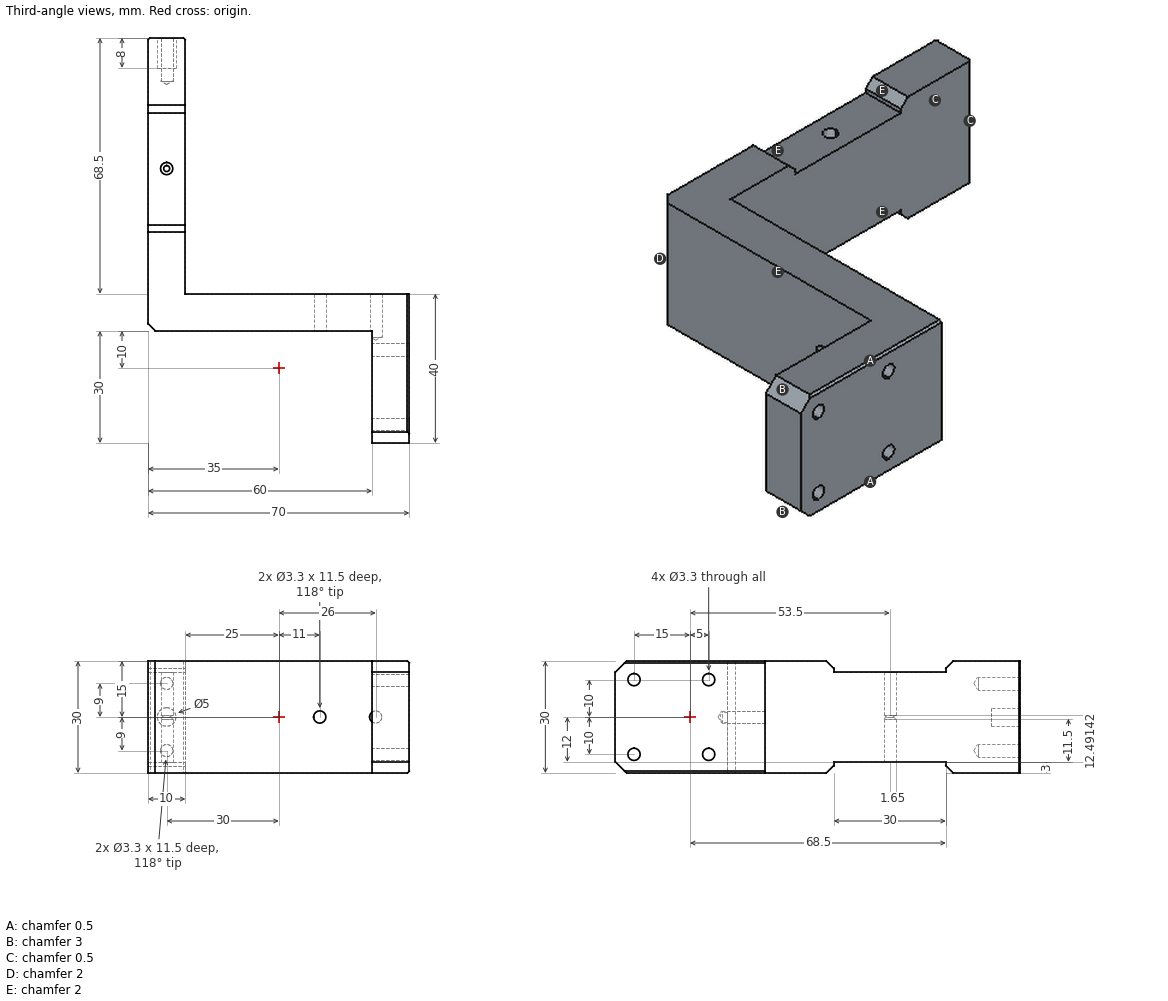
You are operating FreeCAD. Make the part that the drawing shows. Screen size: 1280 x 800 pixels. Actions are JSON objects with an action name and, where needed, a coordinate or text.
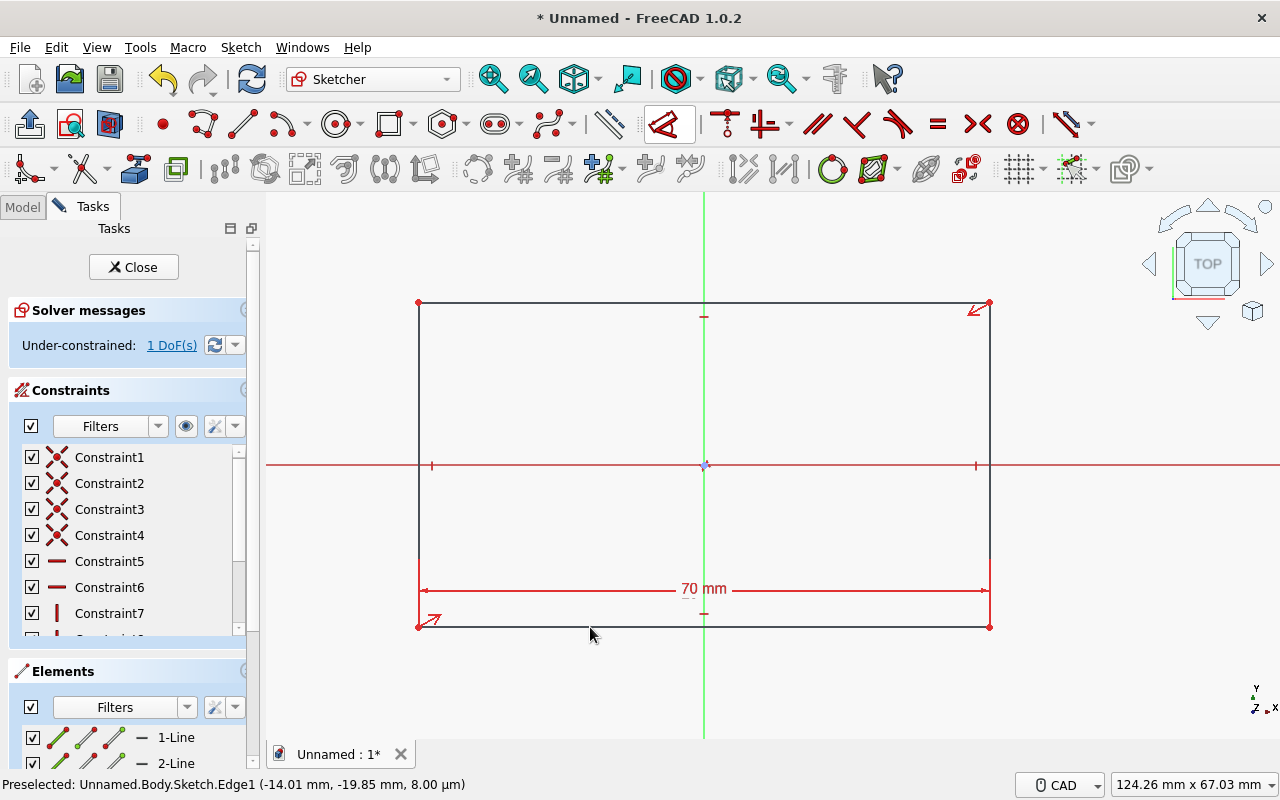
{"action": "left_click", "coordinate": [990, 530]}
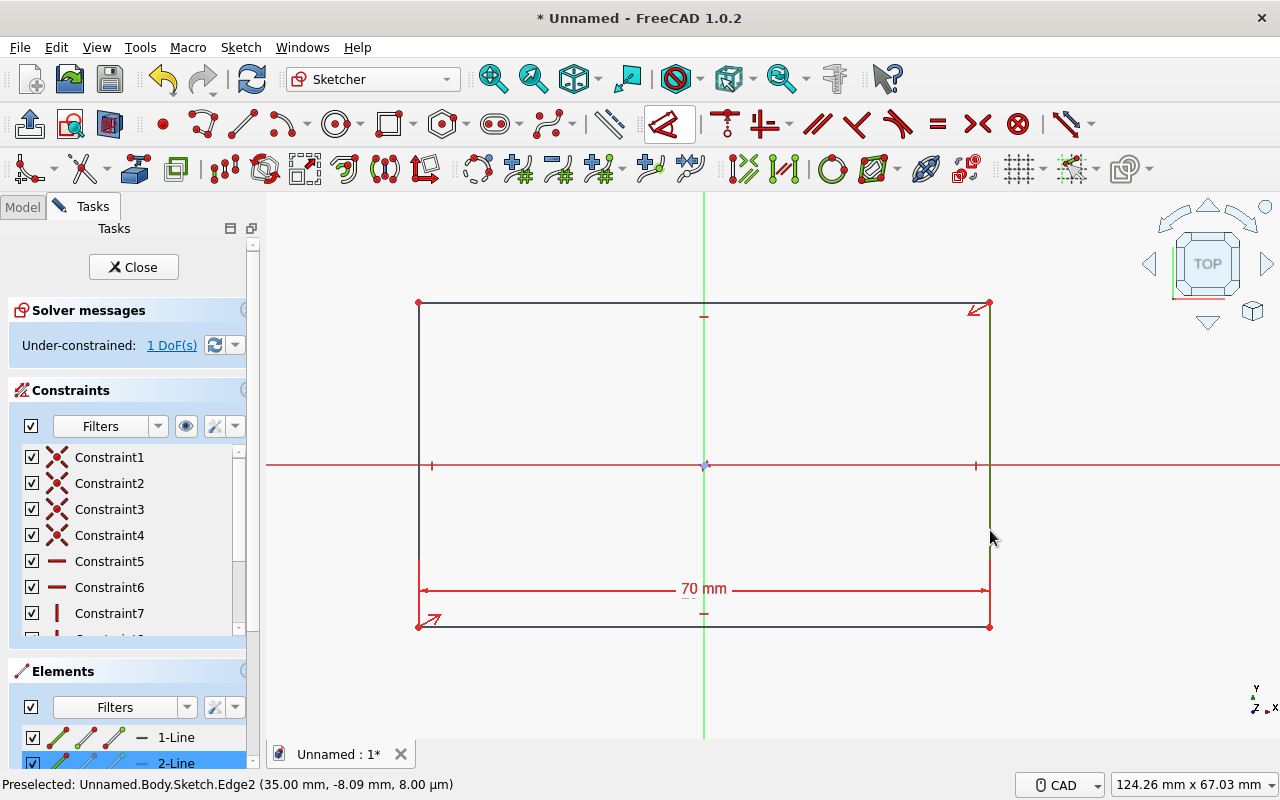
{"action": "key", "text": "i"}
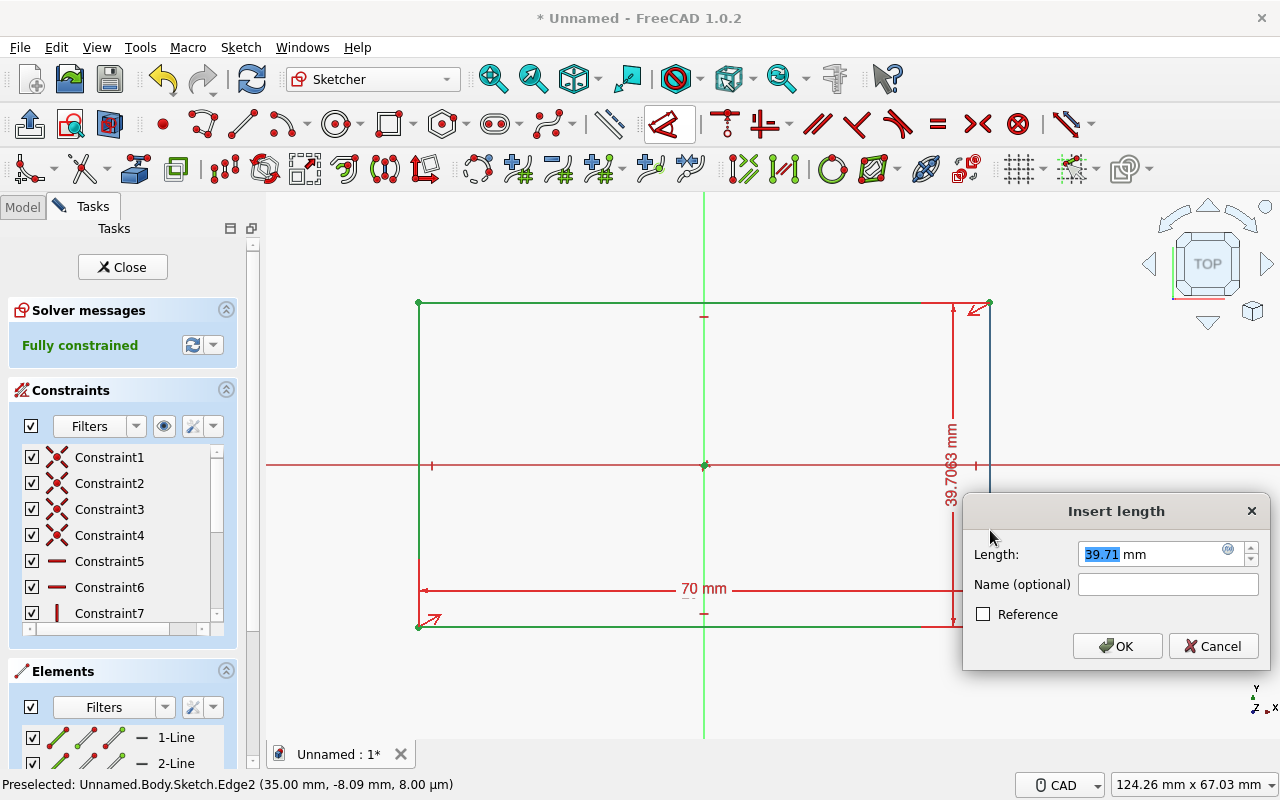
{"action": "type", "text": "40"}
{"action": "key", "text": "Return"}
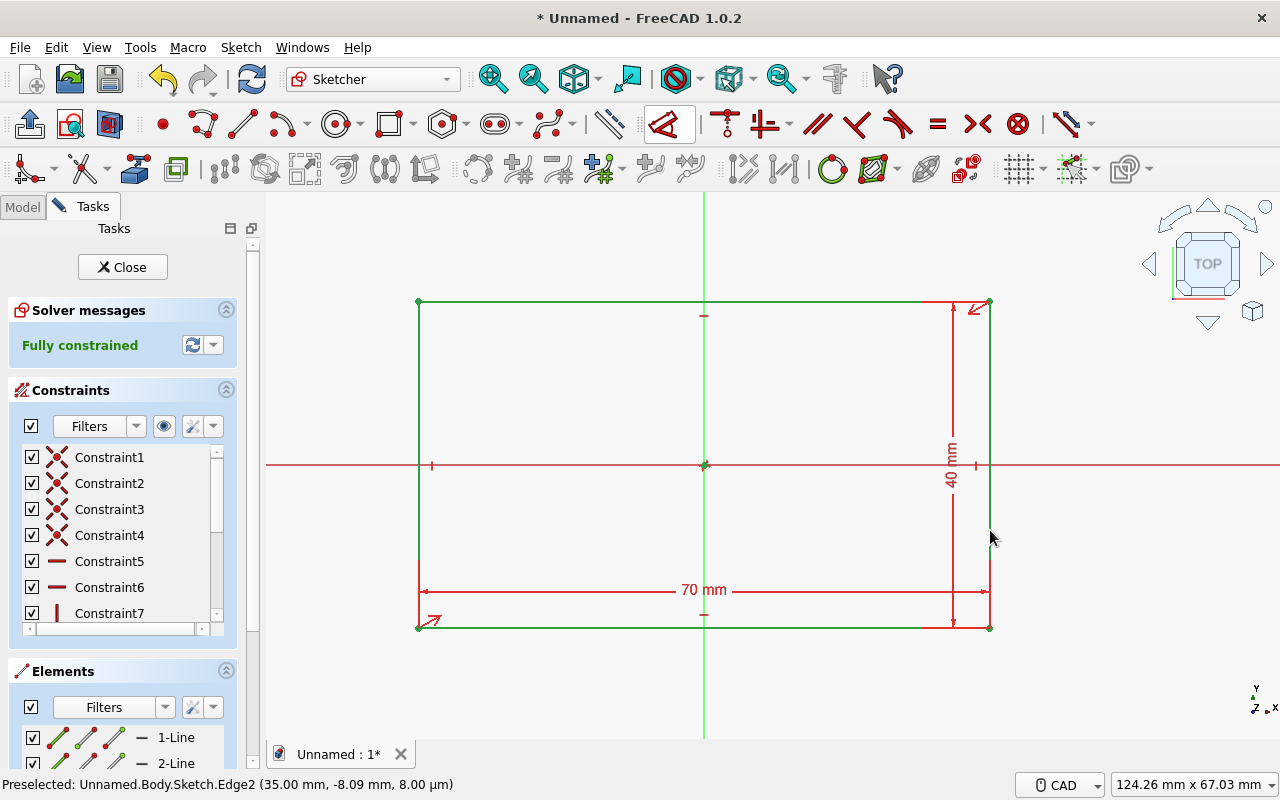
{"action": "left_click", "coordinate": [123, 267]}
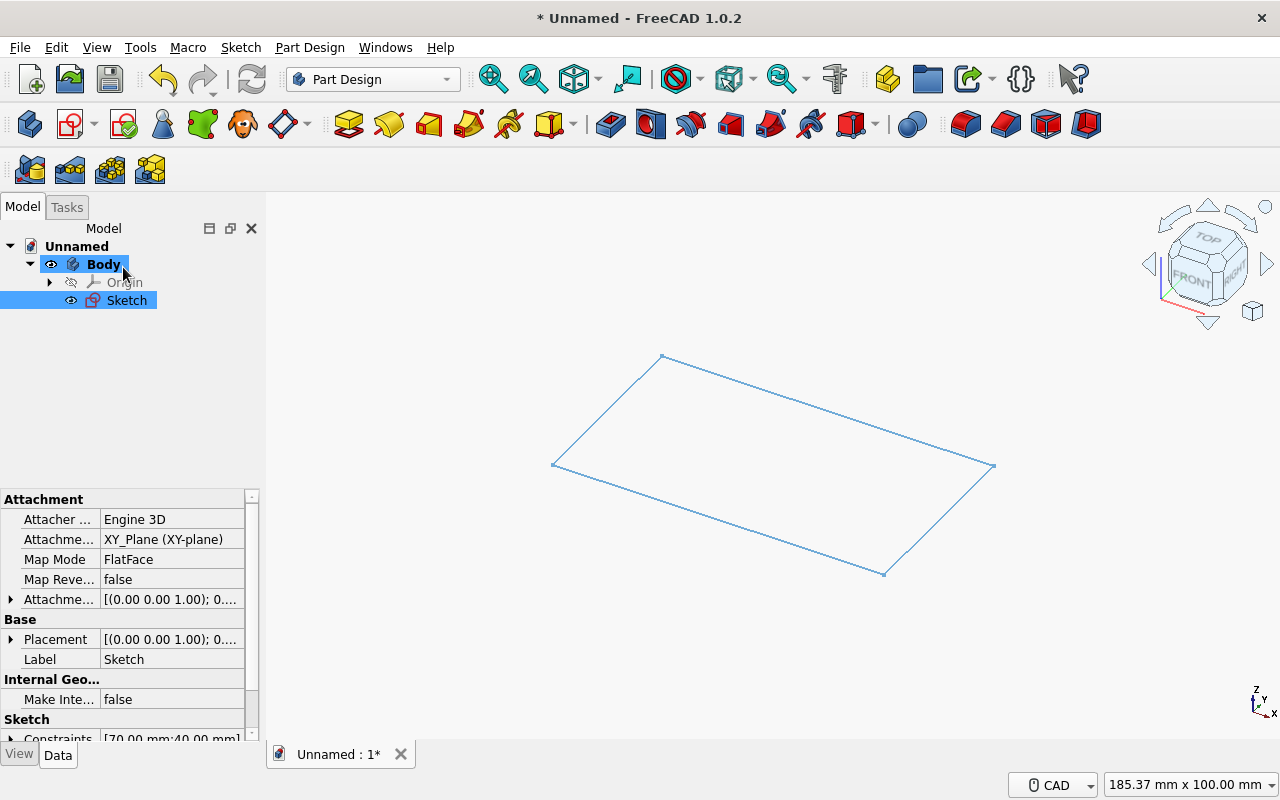
{"action": "left_click", "coordinate": [350, 124]}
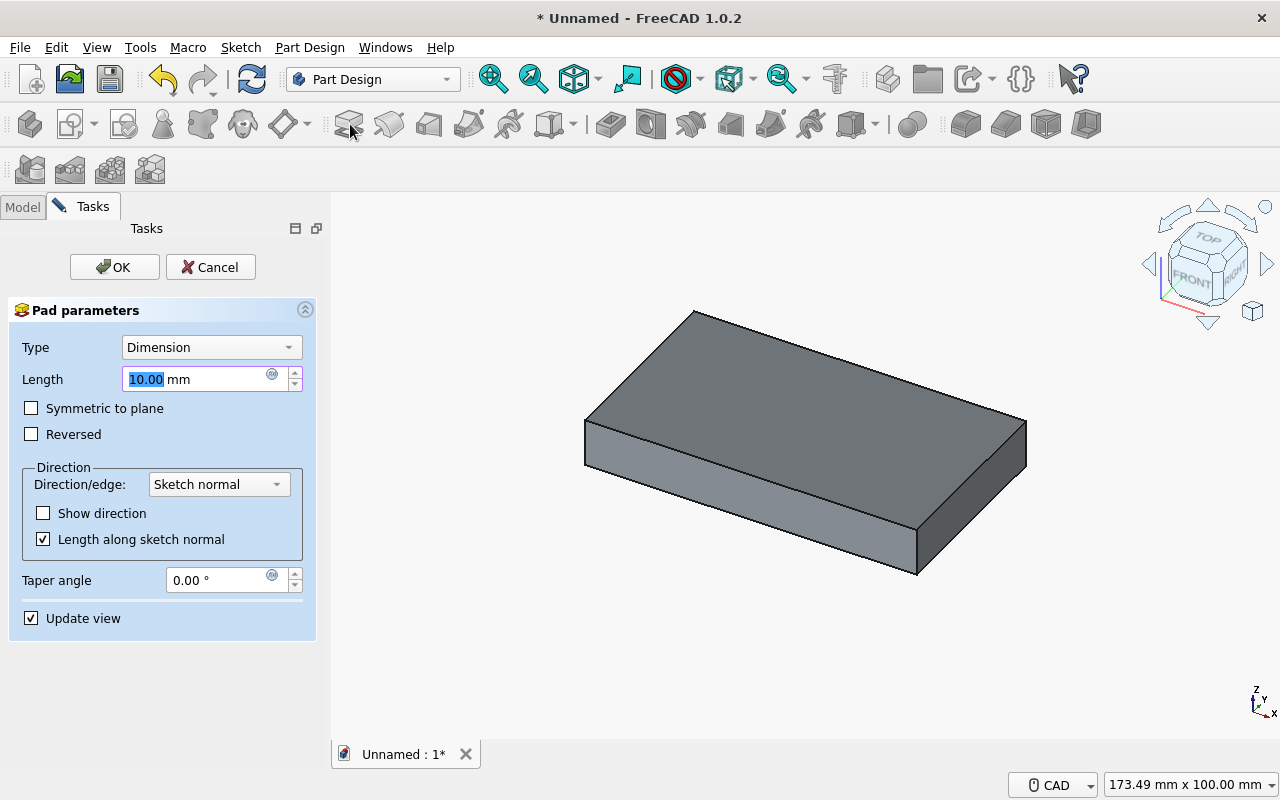
{"action": "type", "text": "30"}
{"action": "key", "text": "Tab"}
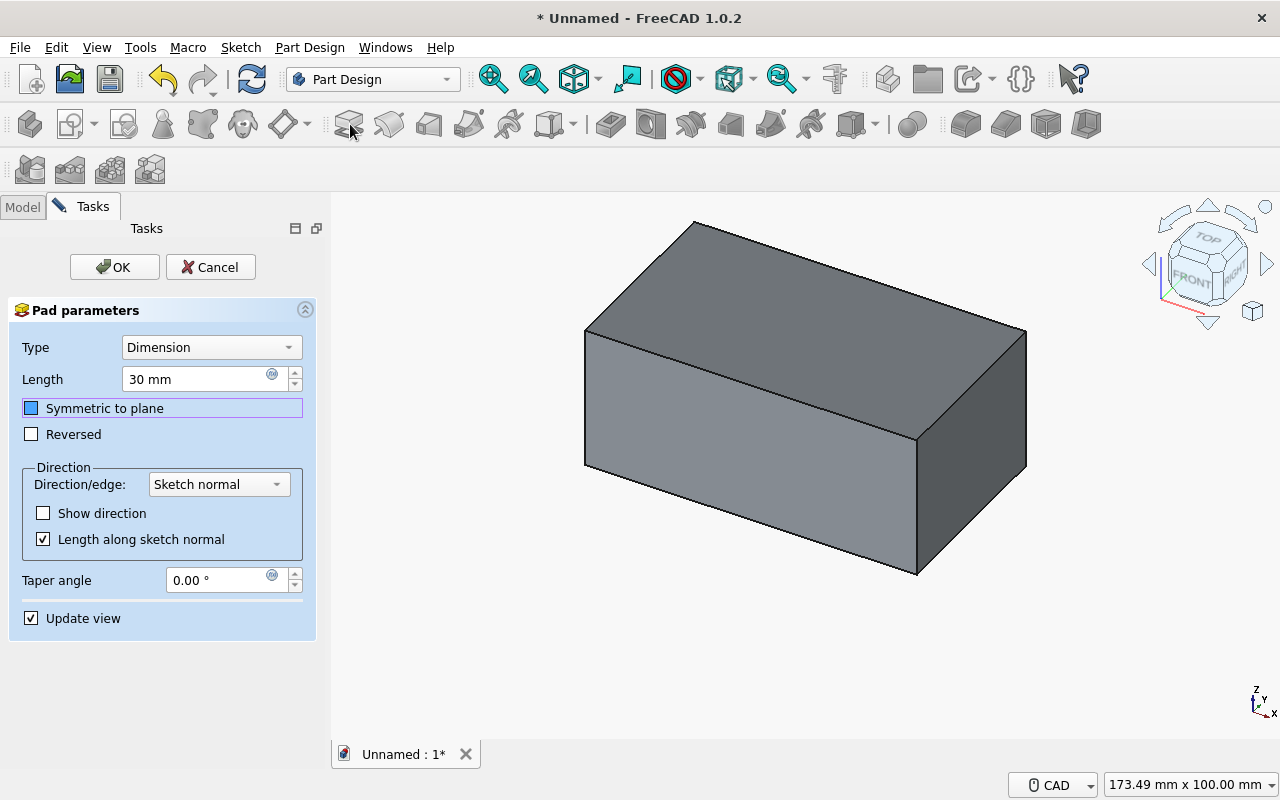
{"action": "left_click", "coordinate": [30, 408]}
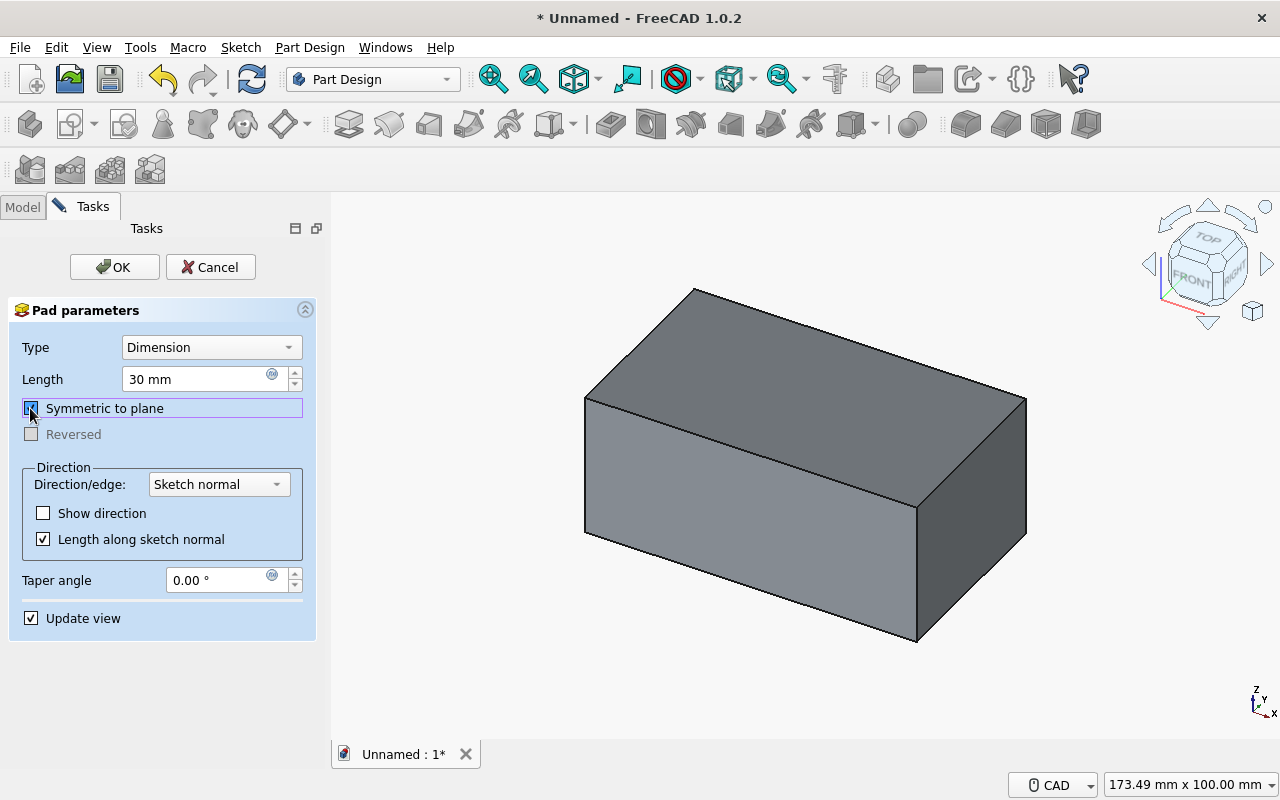
{"action": "left_click", "coordinate": [115, 267]}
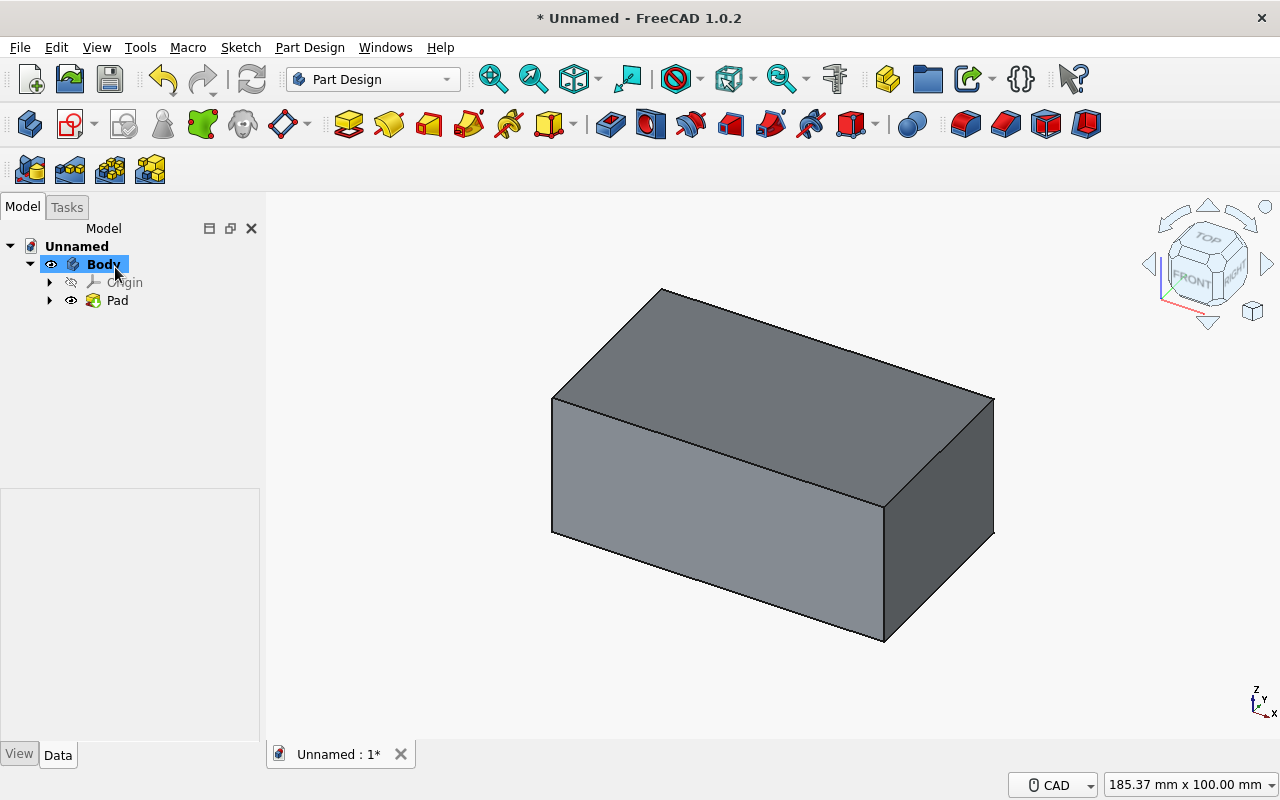
{"action": "left_click", "coordinate": [820, 413]}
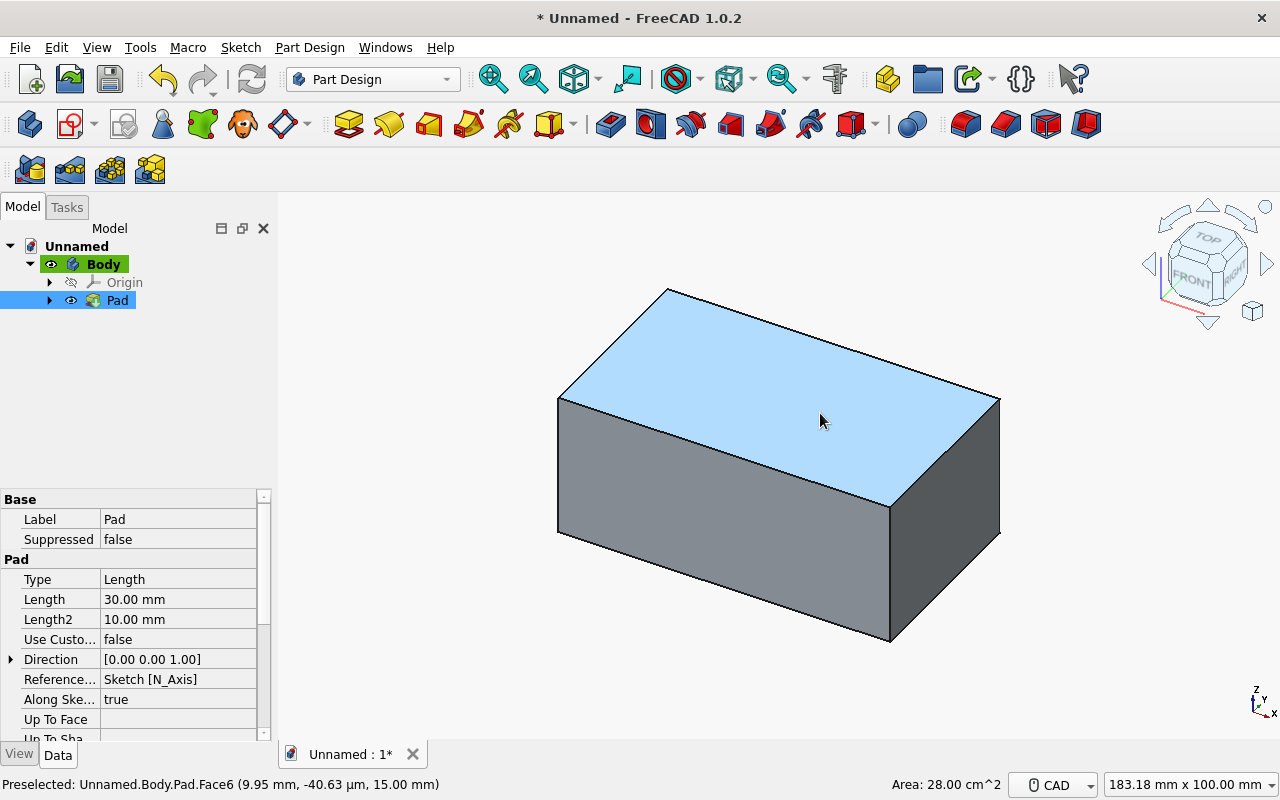
{"action": "left_click", "coordinate": [70, 124]}